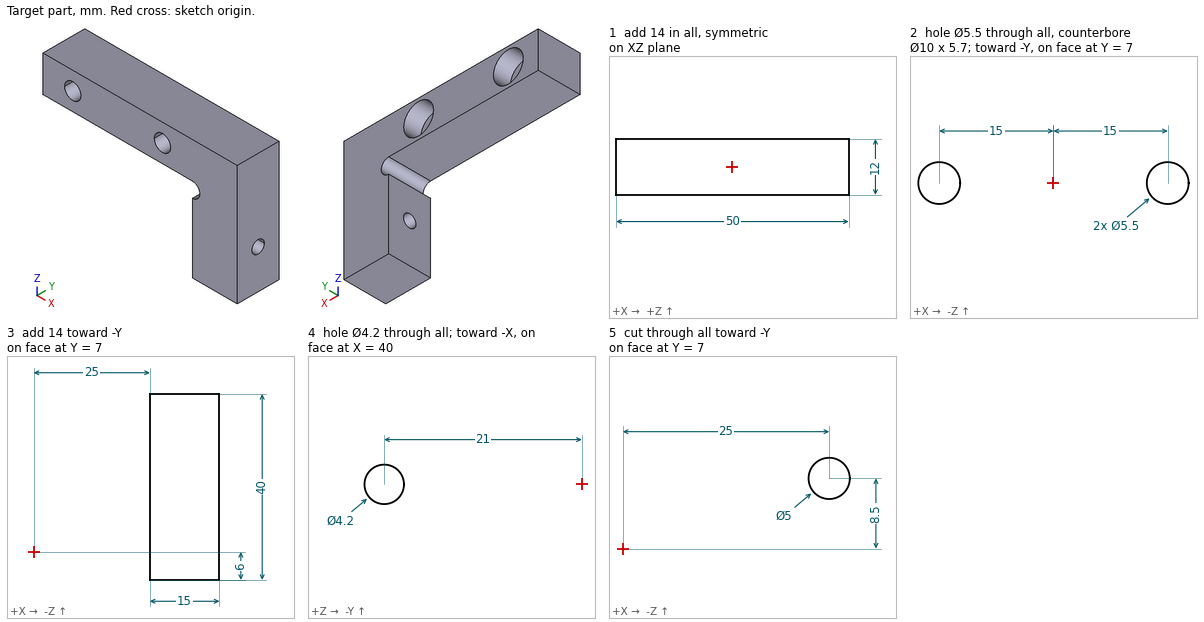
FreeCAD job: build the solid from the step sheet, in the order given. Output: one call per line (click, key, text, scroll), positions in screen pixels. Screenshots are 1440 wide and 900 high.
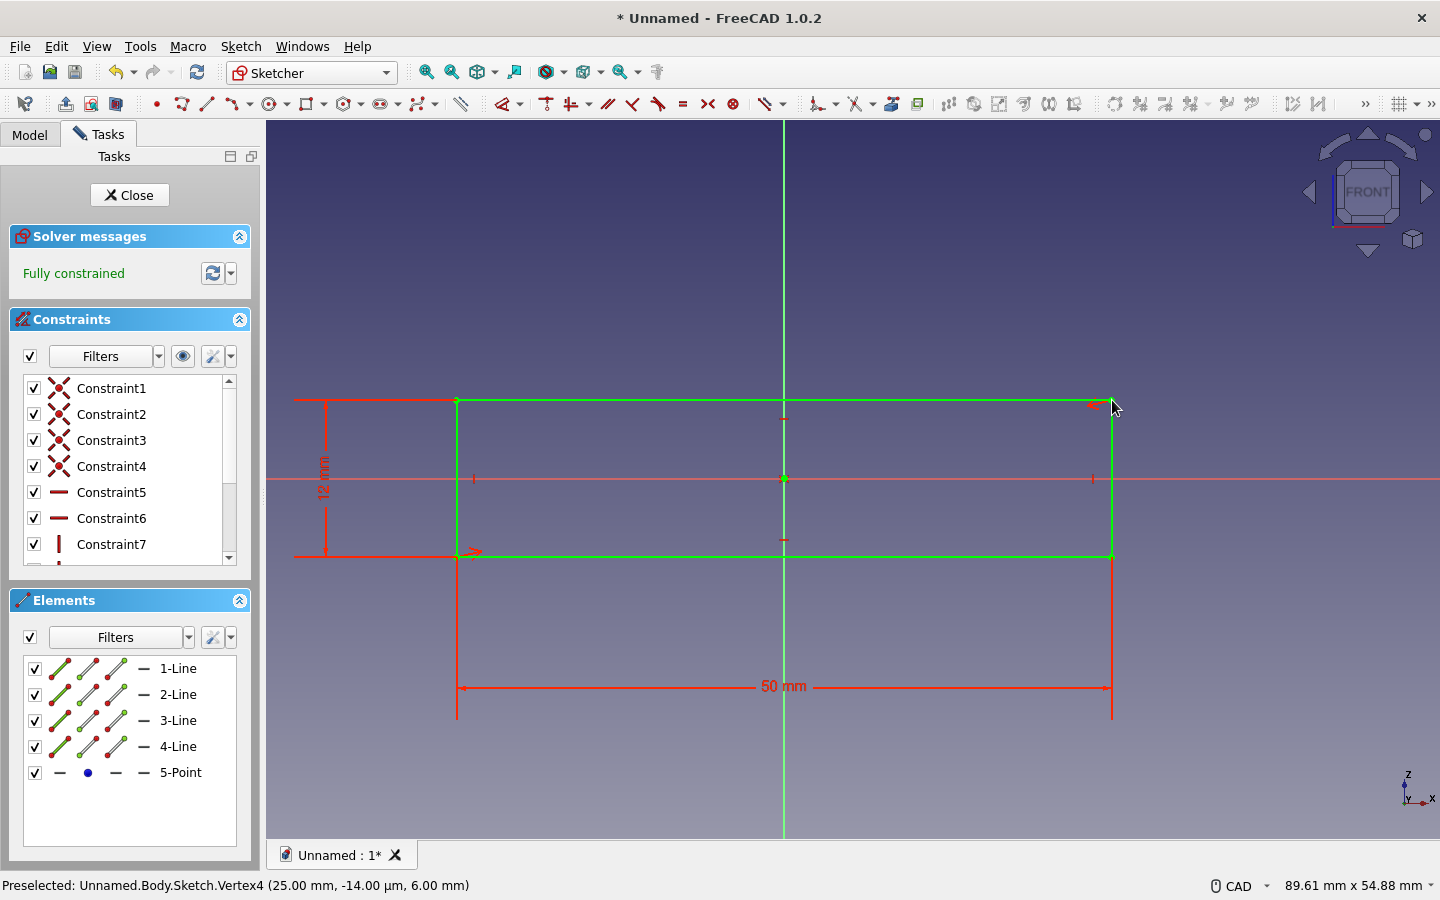
click(130, 195)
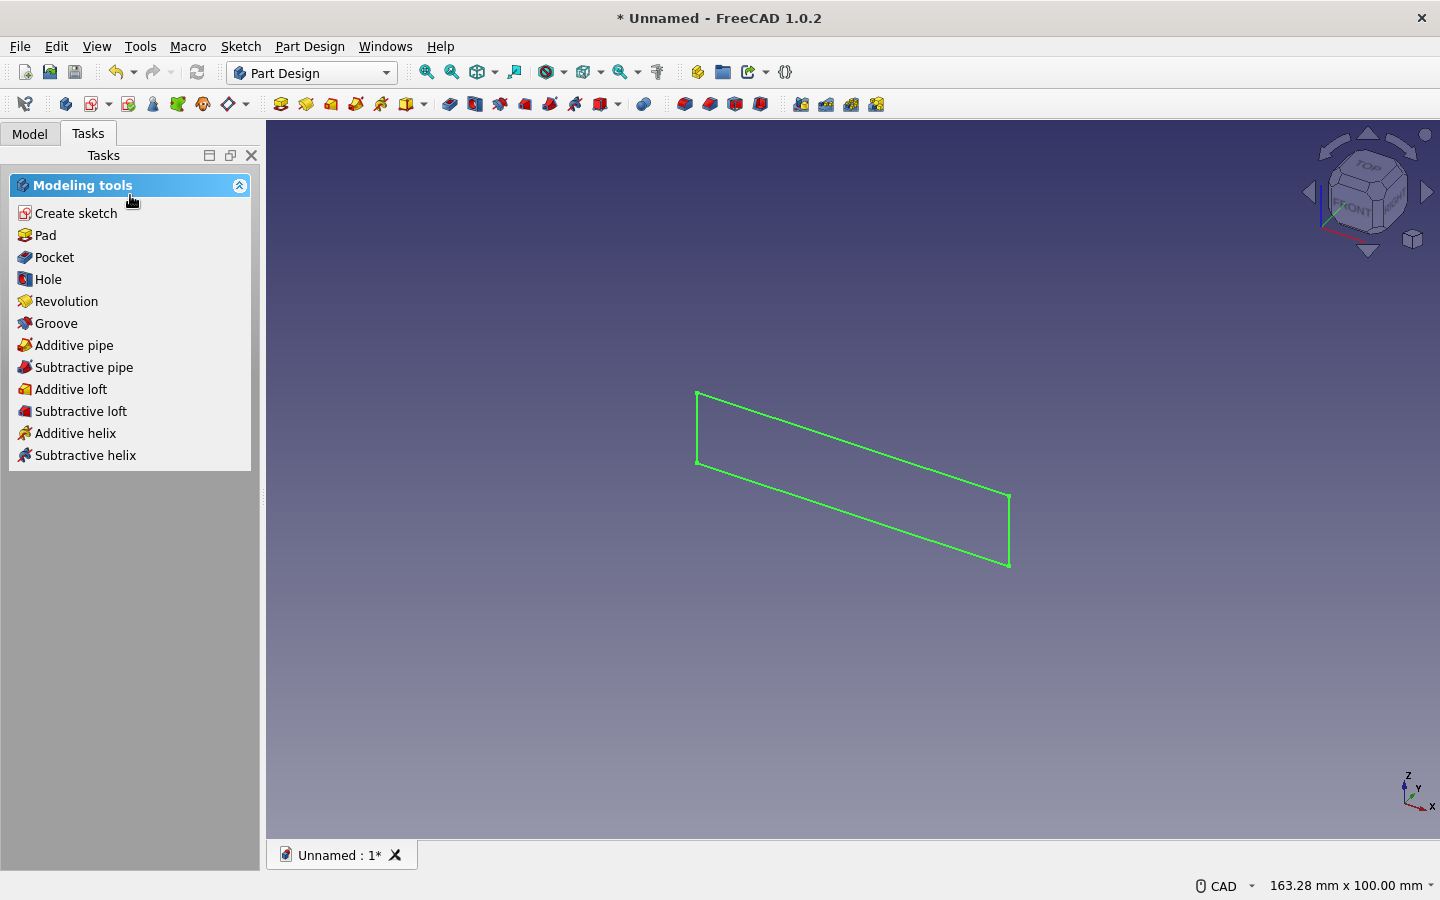
click(281, 104)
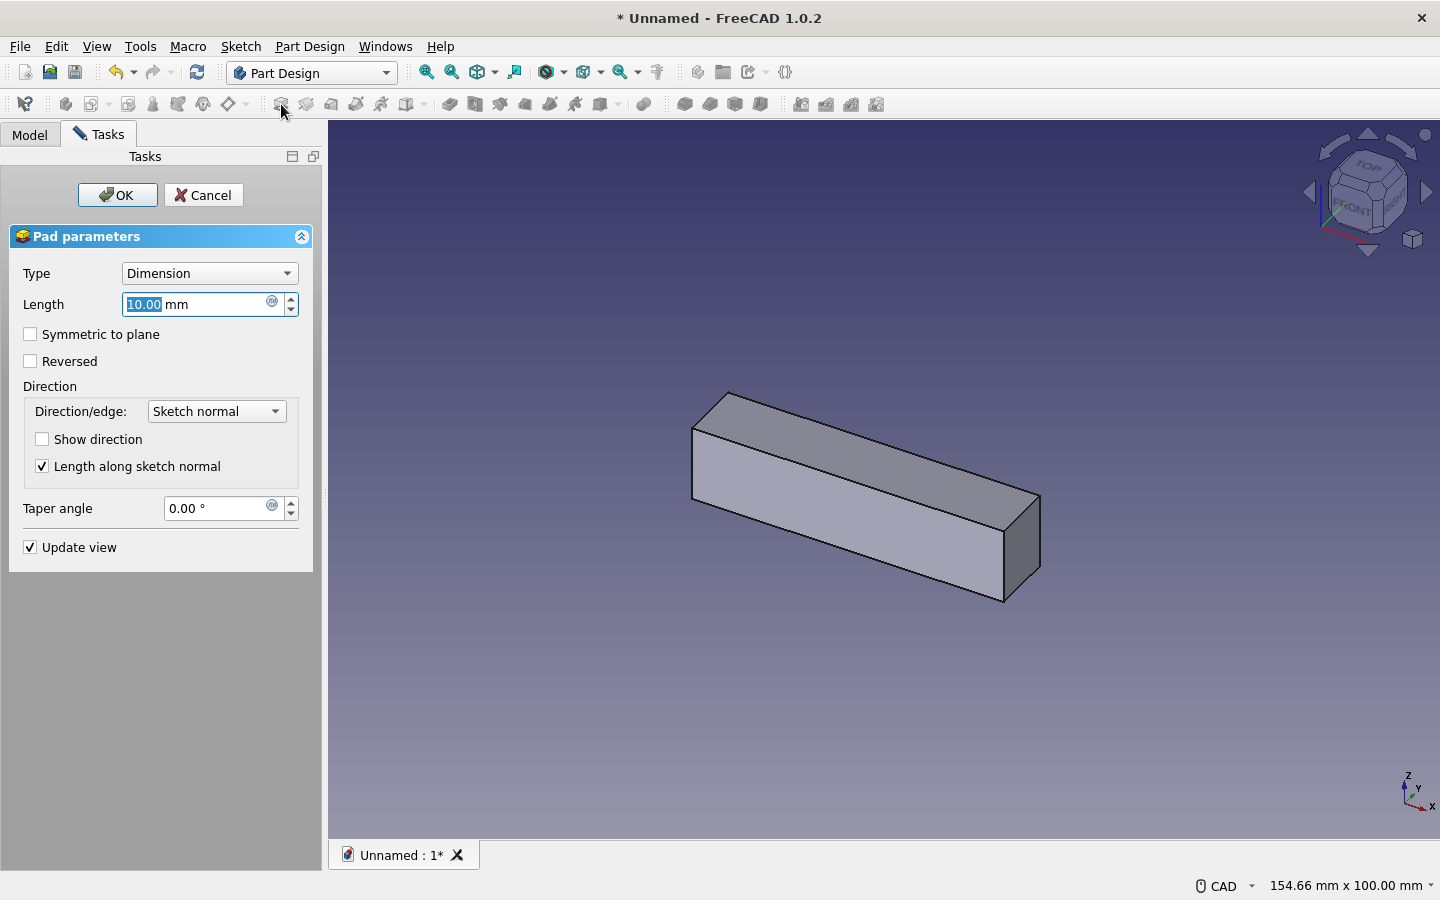
text(14)
key(Tab)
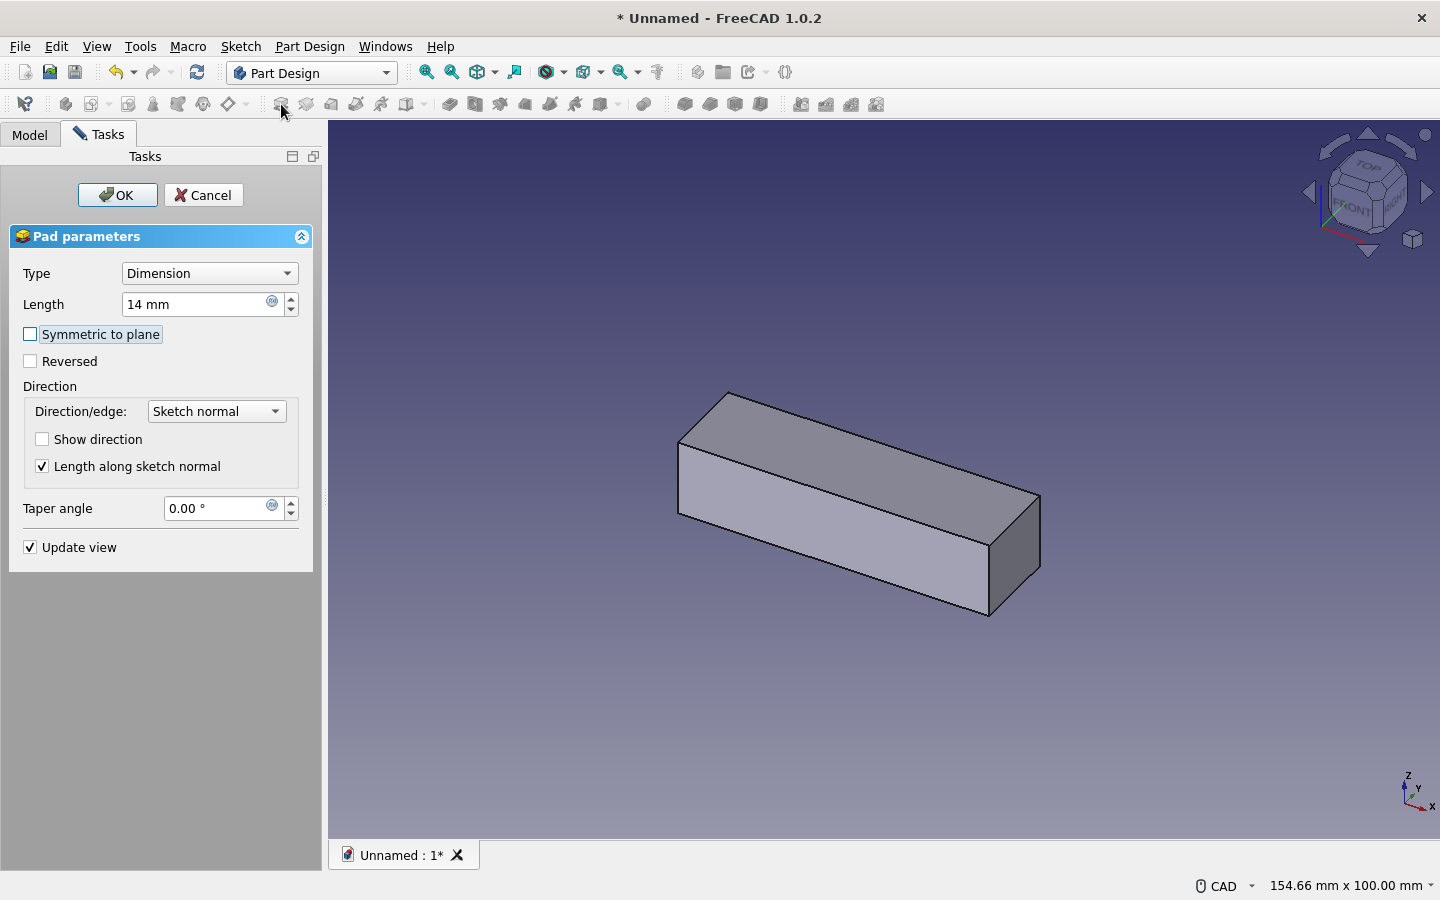
click(31, 334)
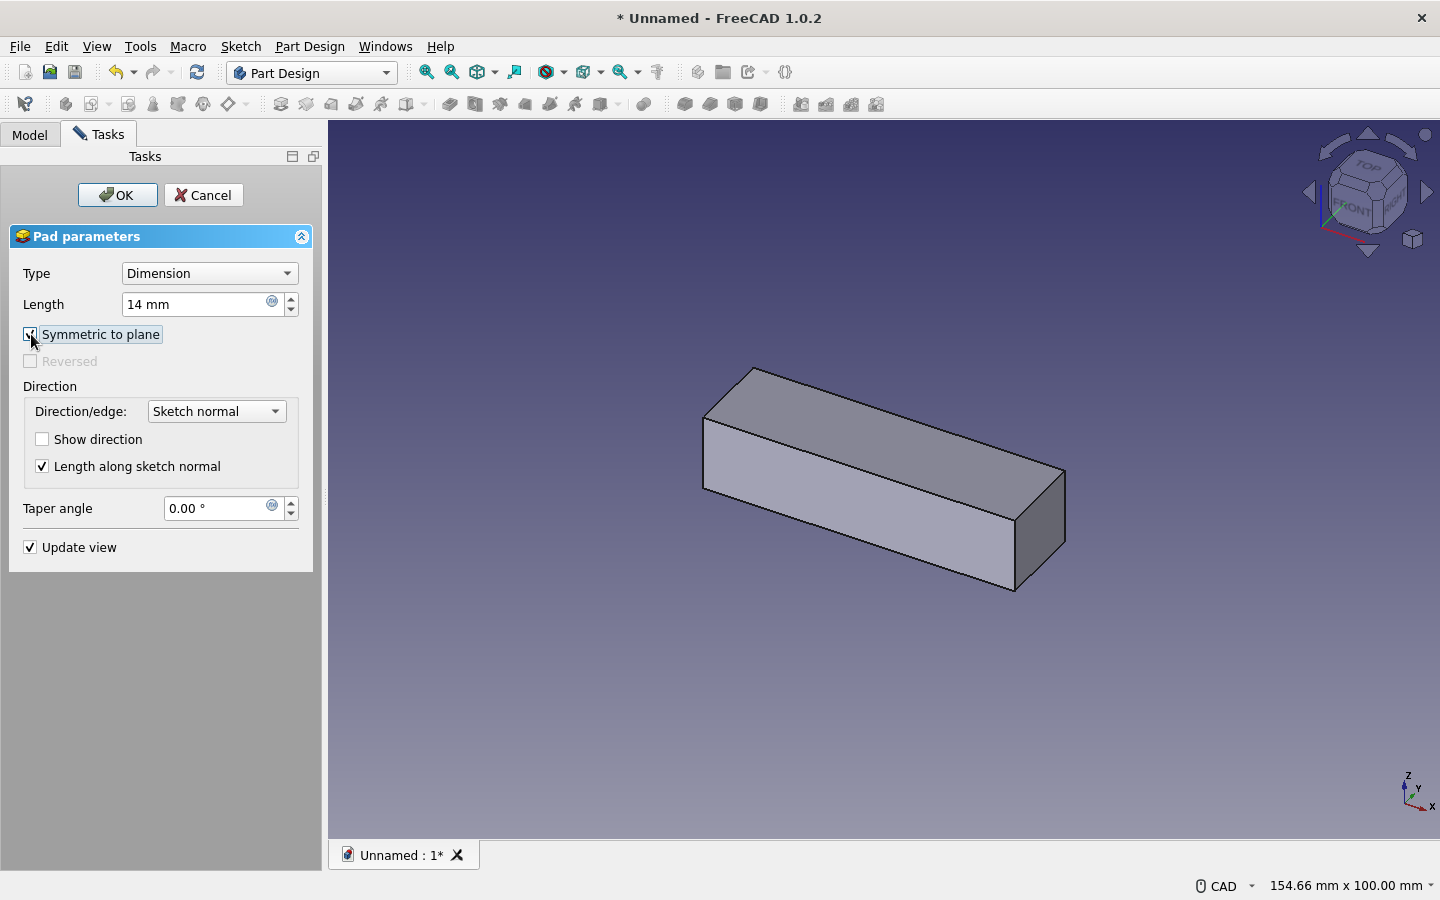
click(118, 195)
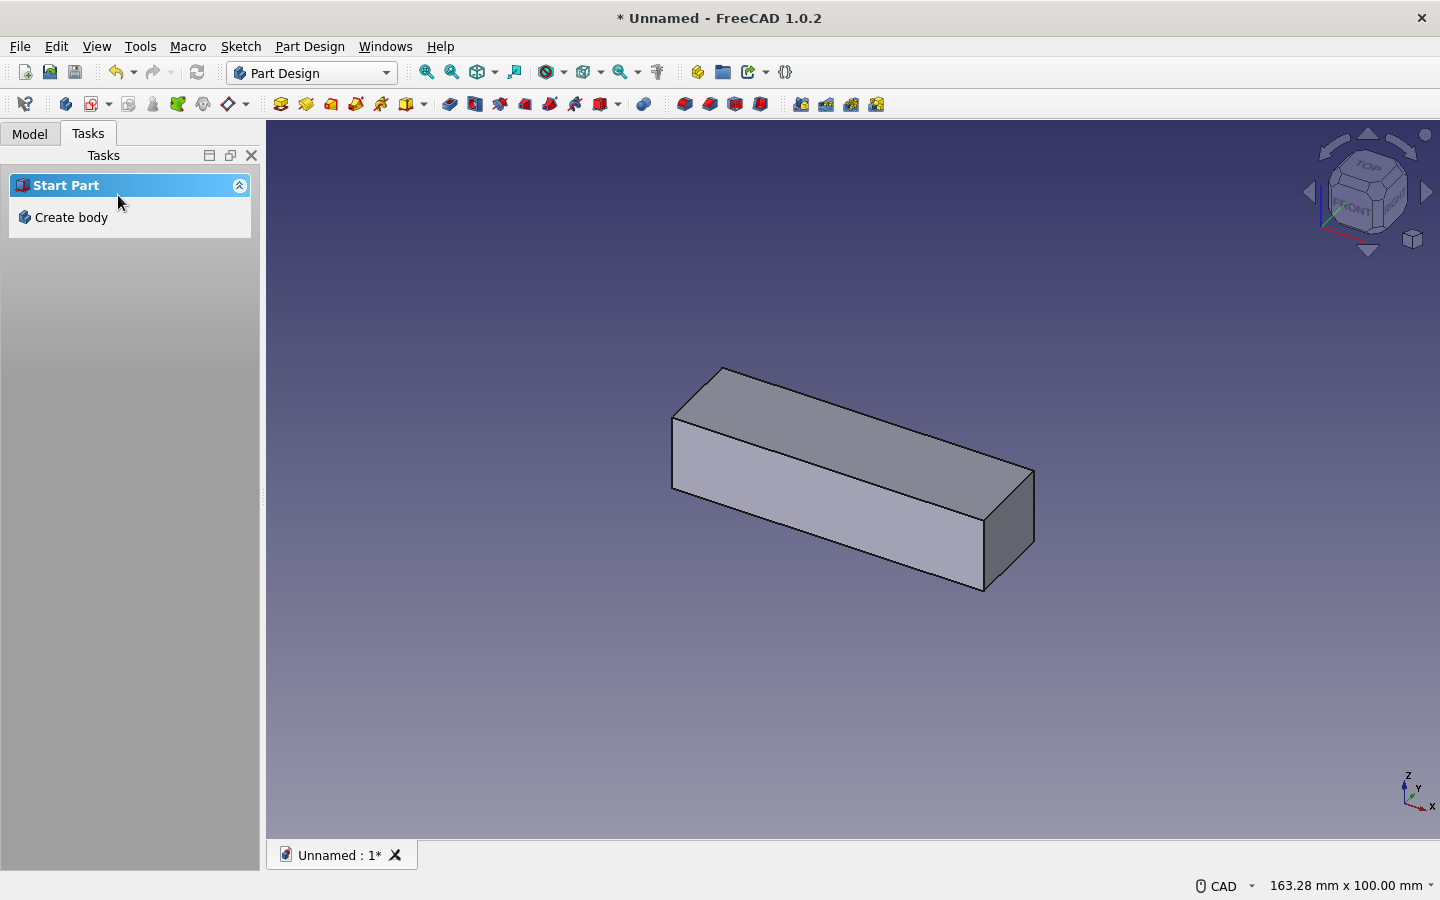
key(v)
key(f)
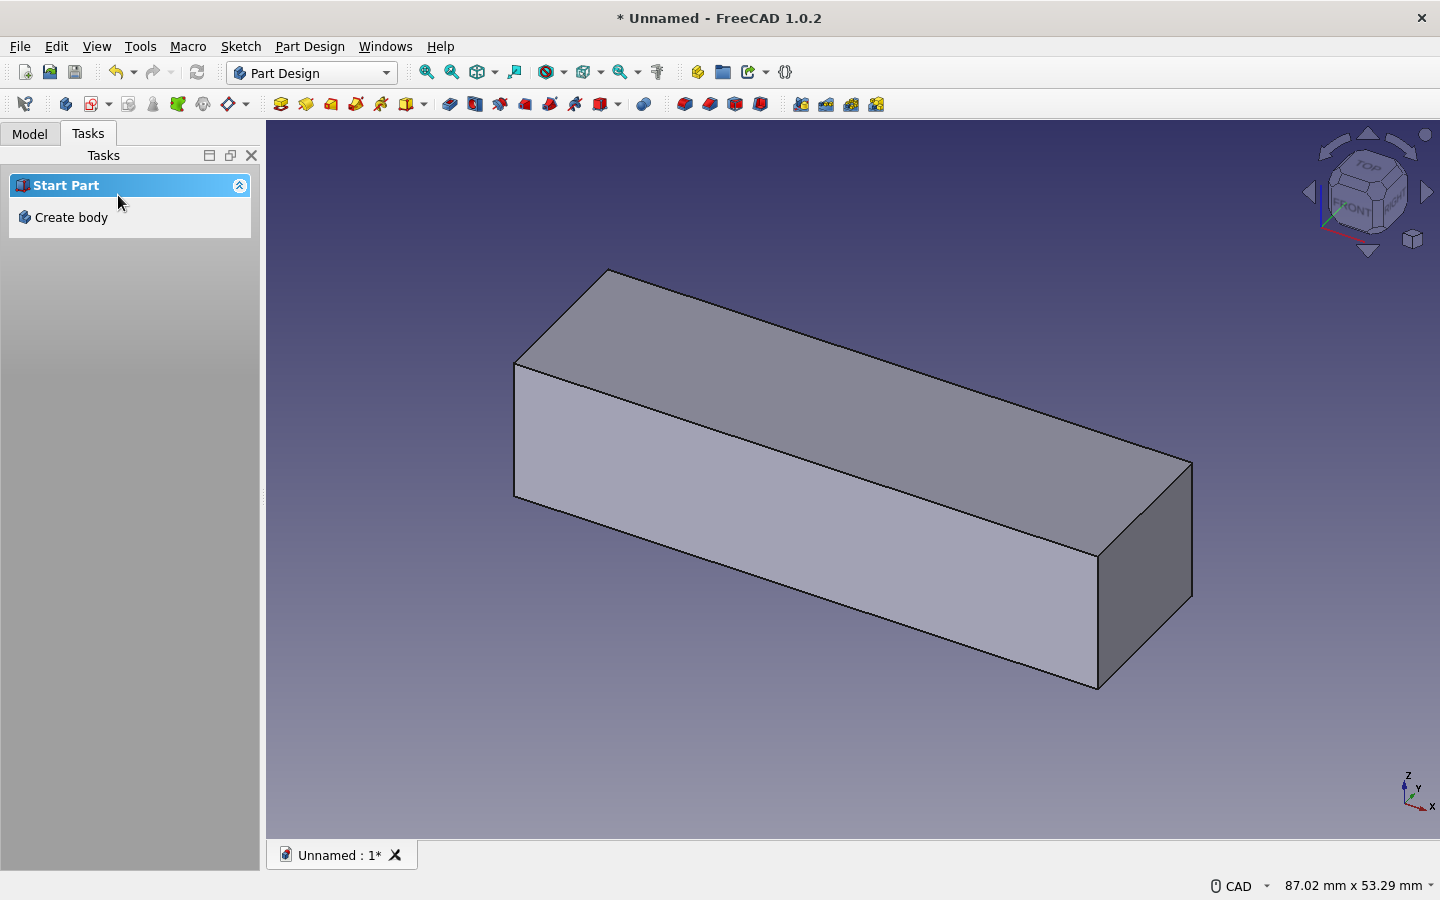
key(4)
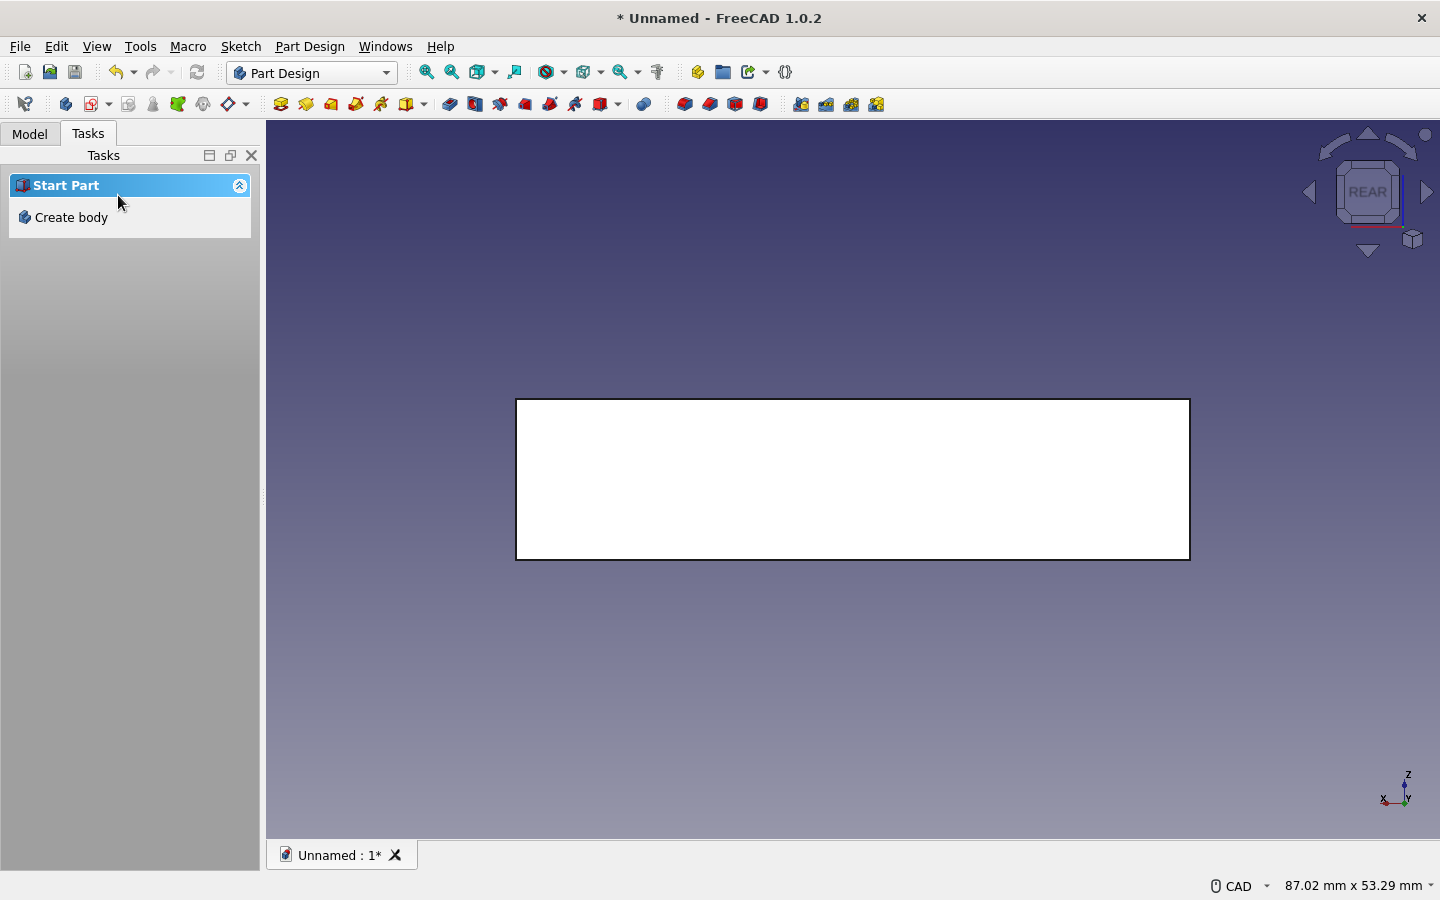
click(660, 479)